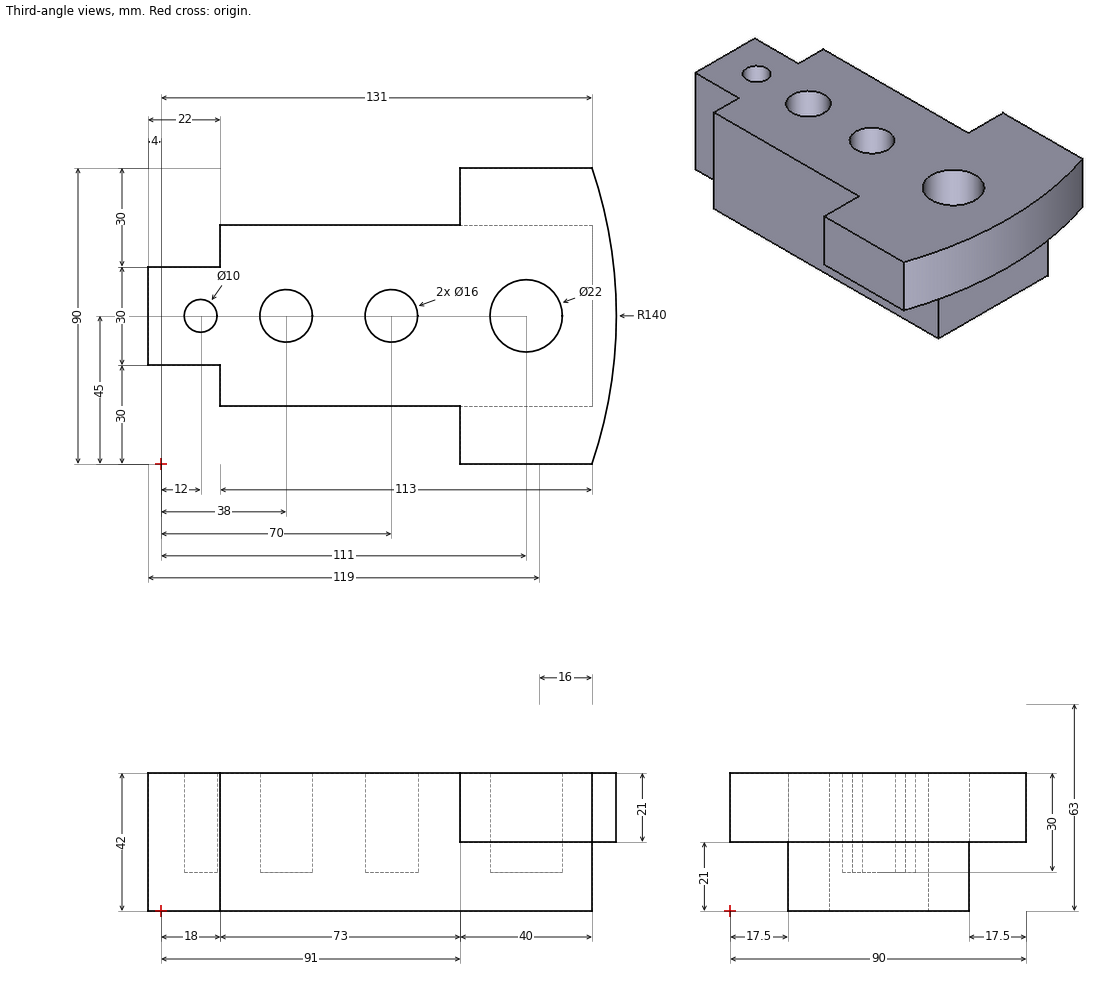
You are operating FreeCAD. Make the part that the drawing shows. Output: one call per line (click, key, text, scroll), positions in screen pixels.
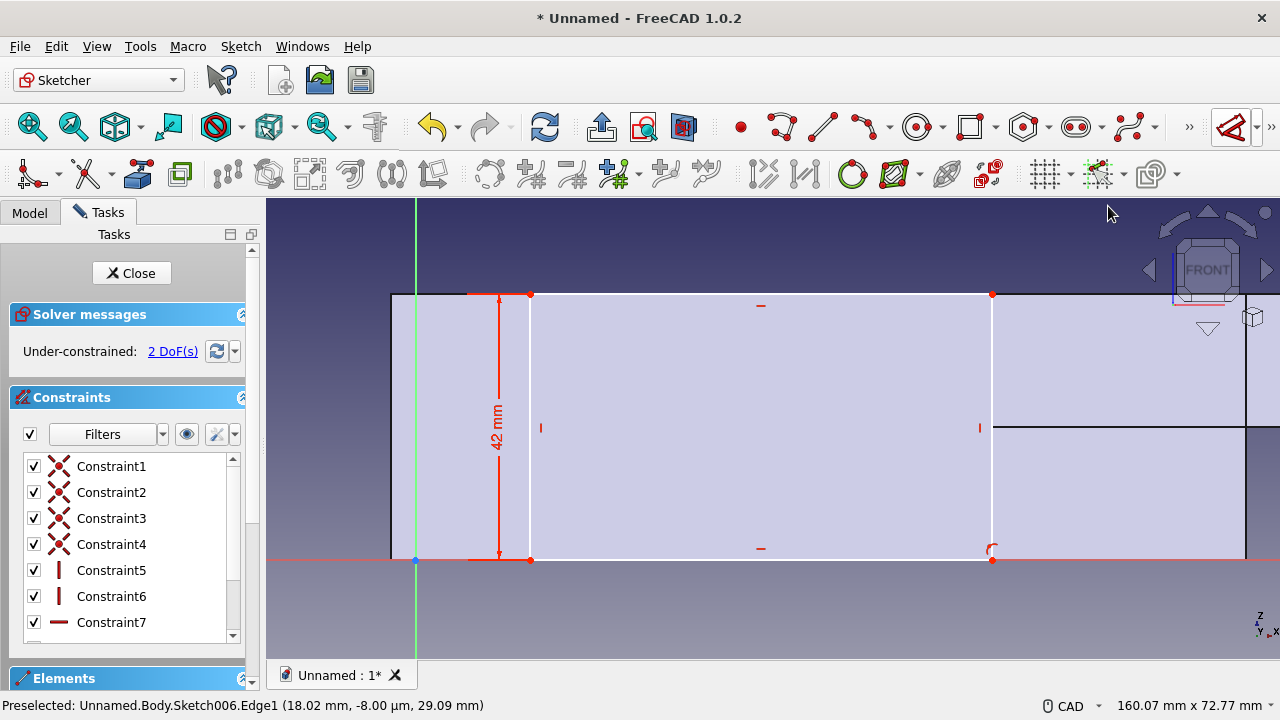
click(669, 560)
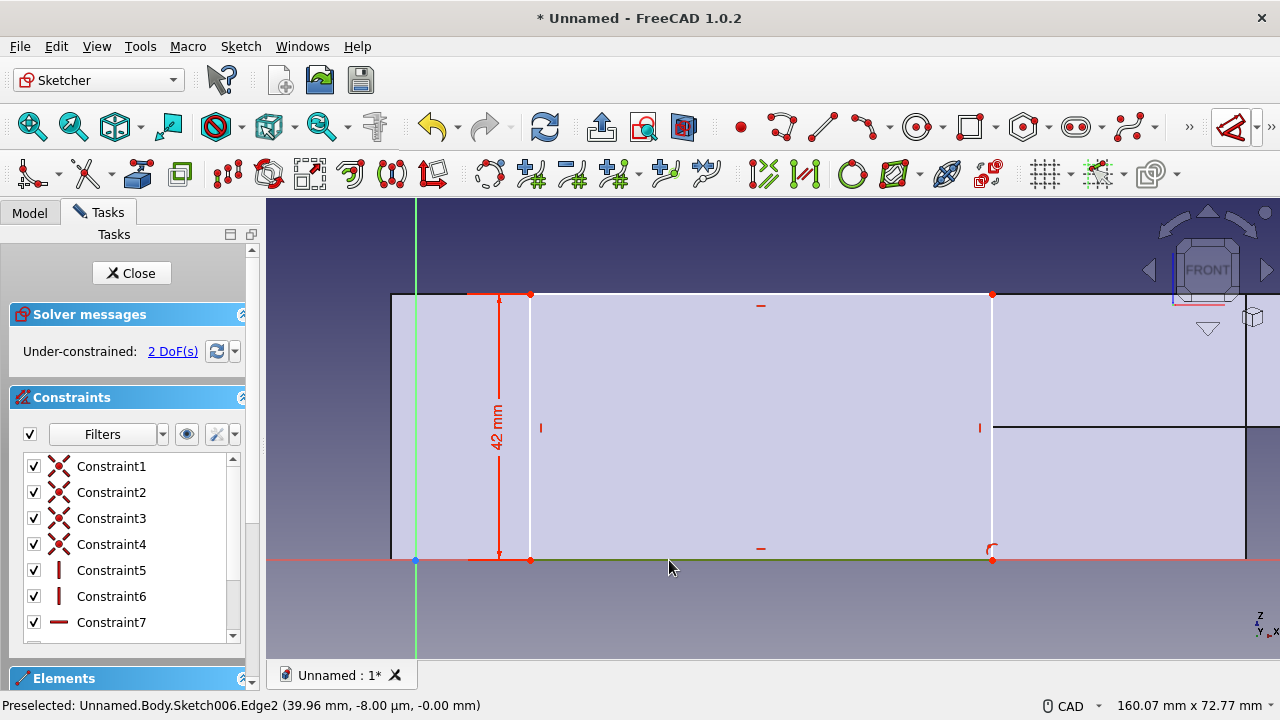
key(l)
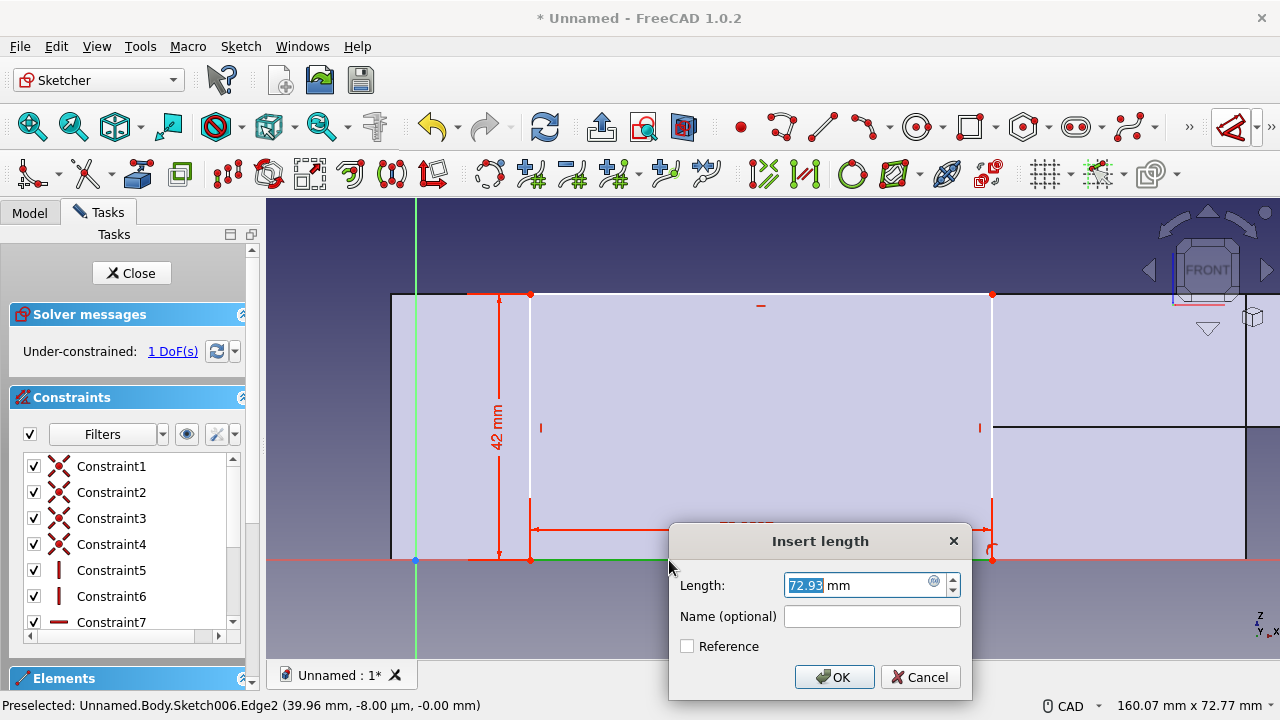
text(73)
key(Return)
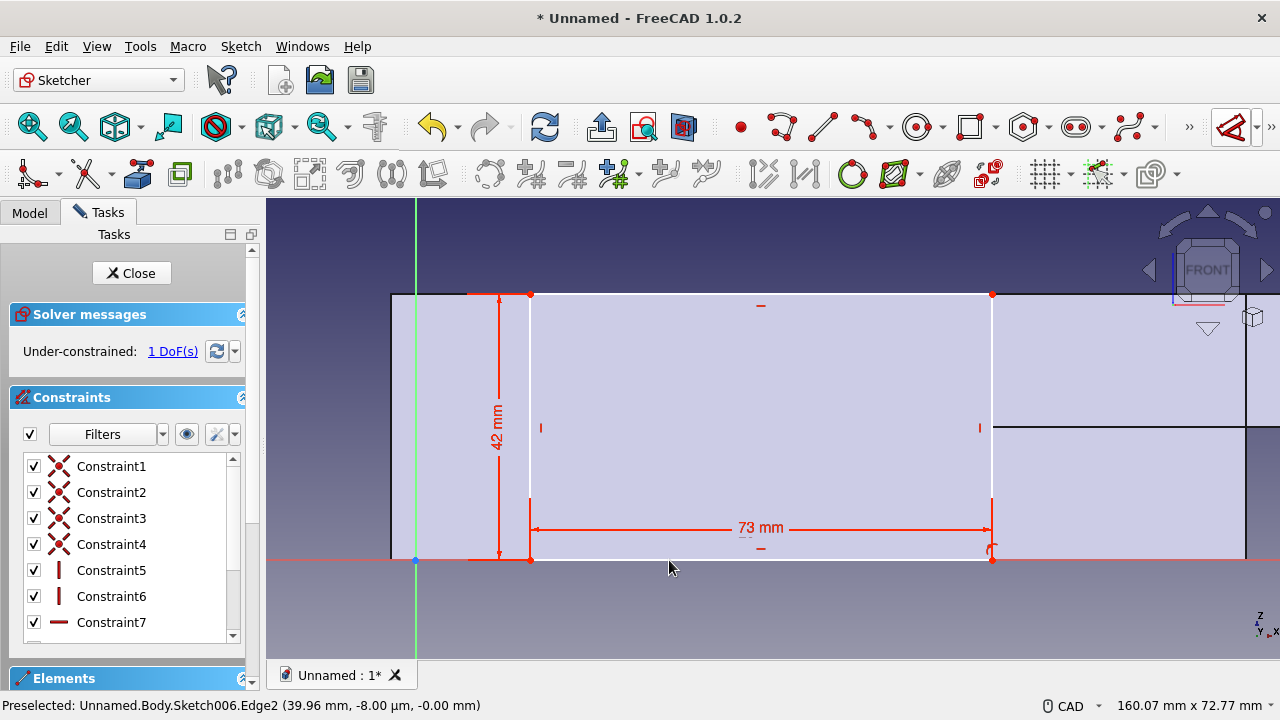
click(530, 294)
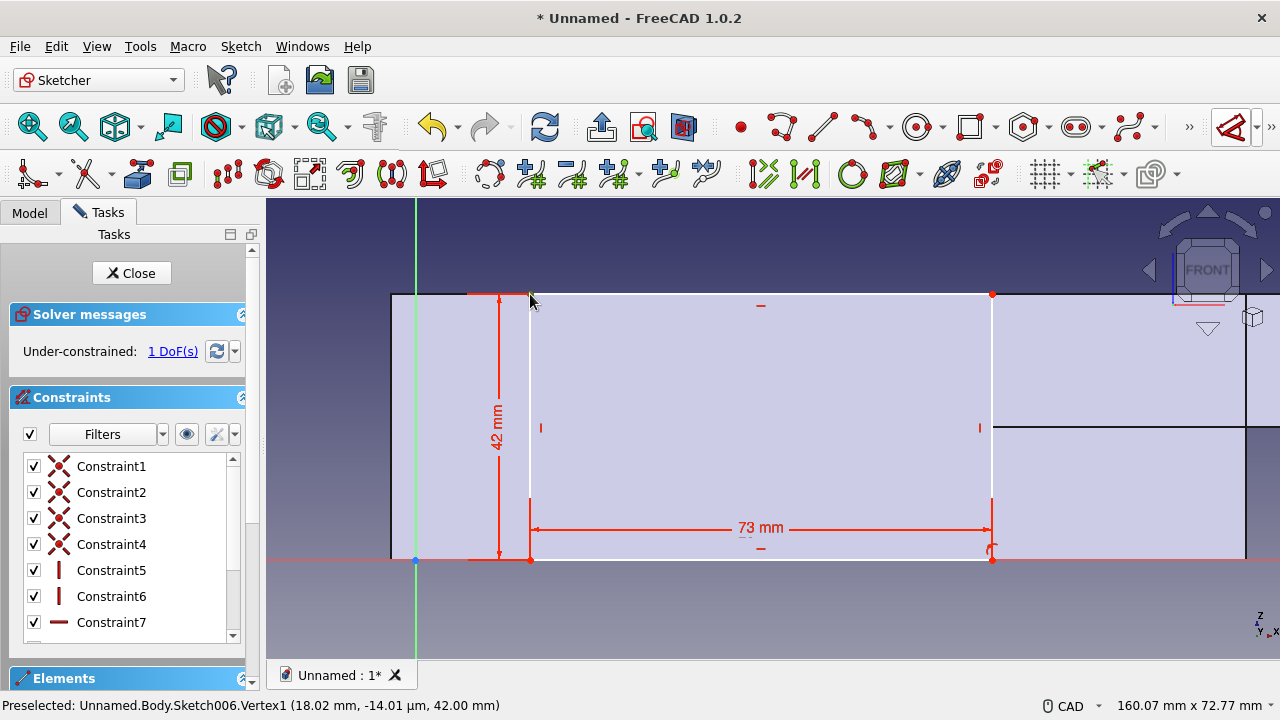
click(1256, 128)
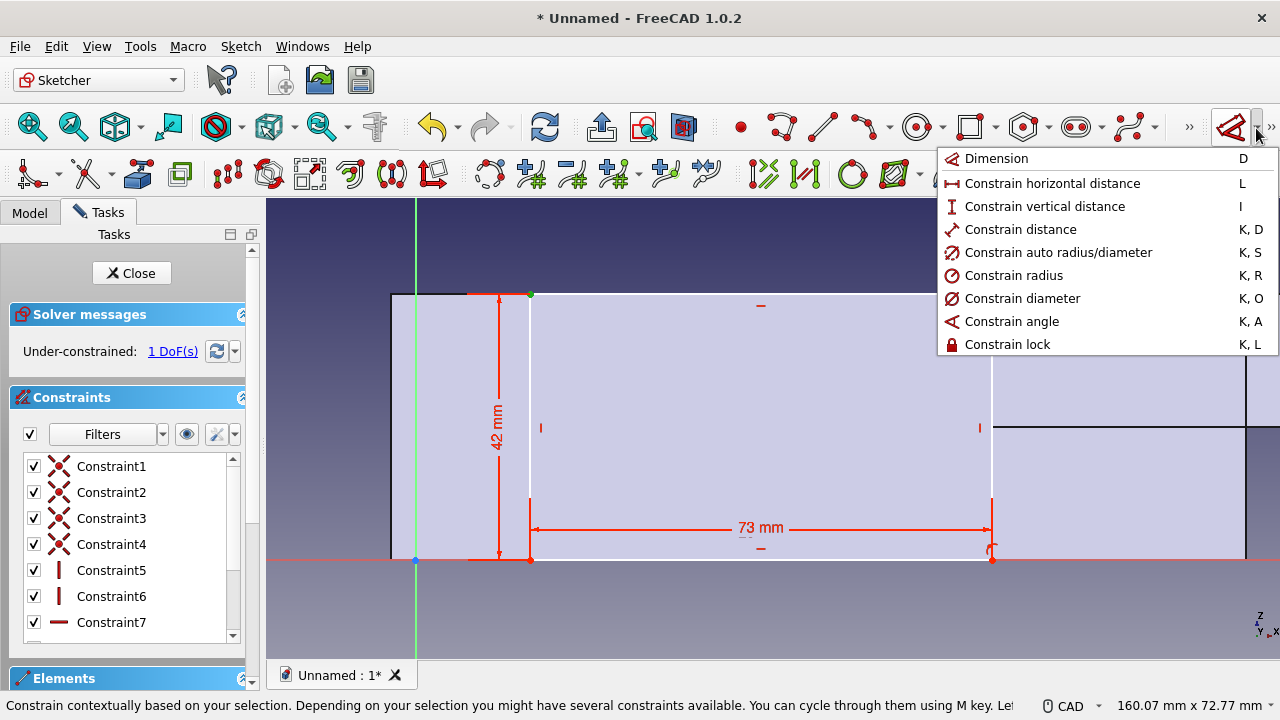
click(1108, 184)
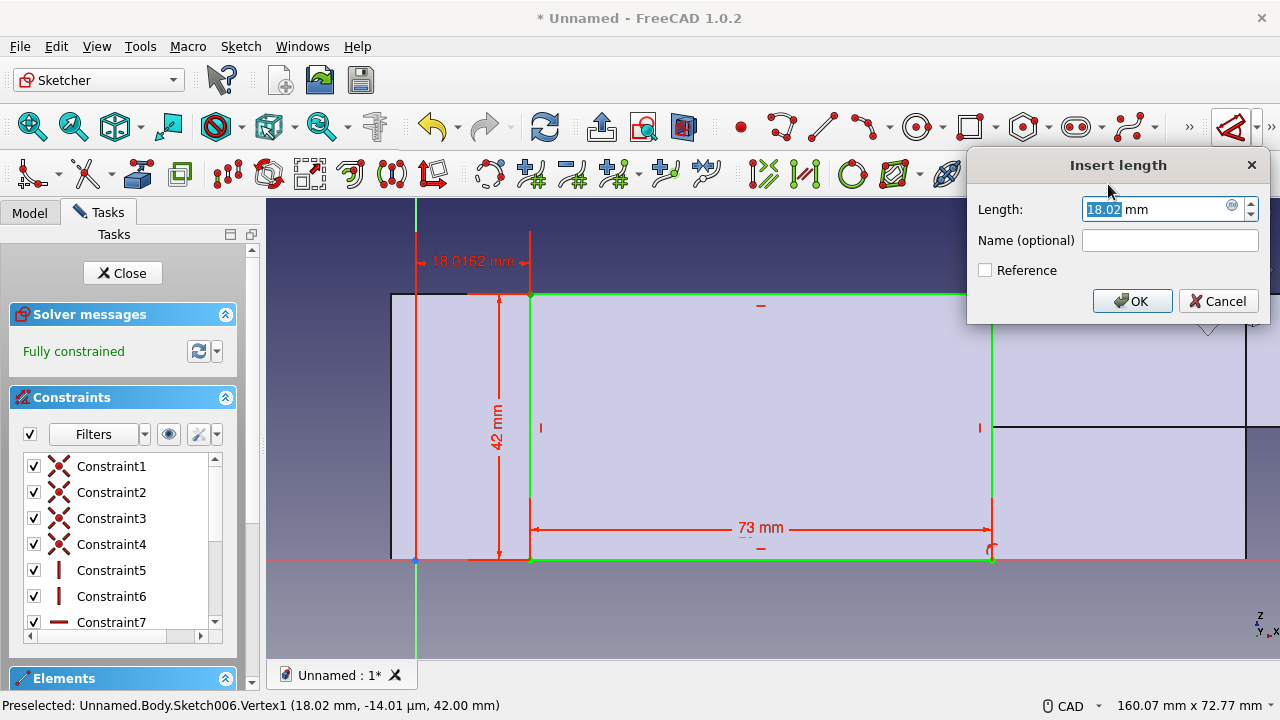
text(18)
key(Return)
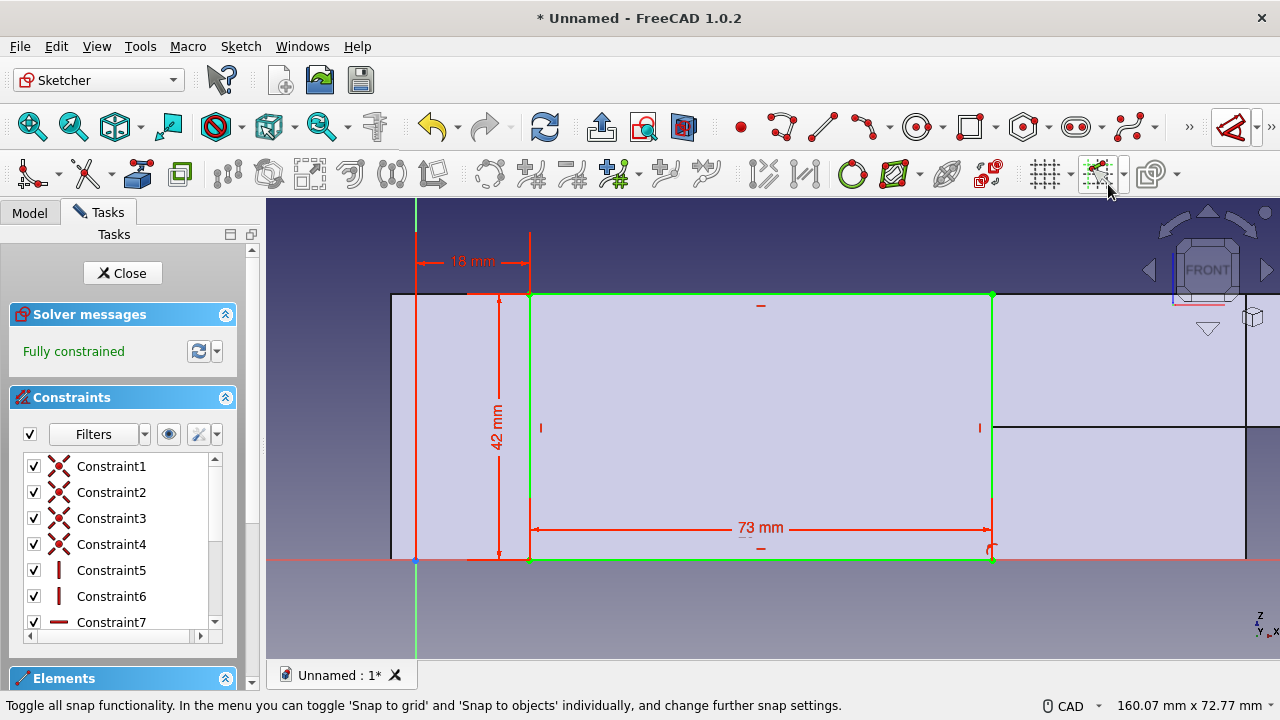
click(123, 273)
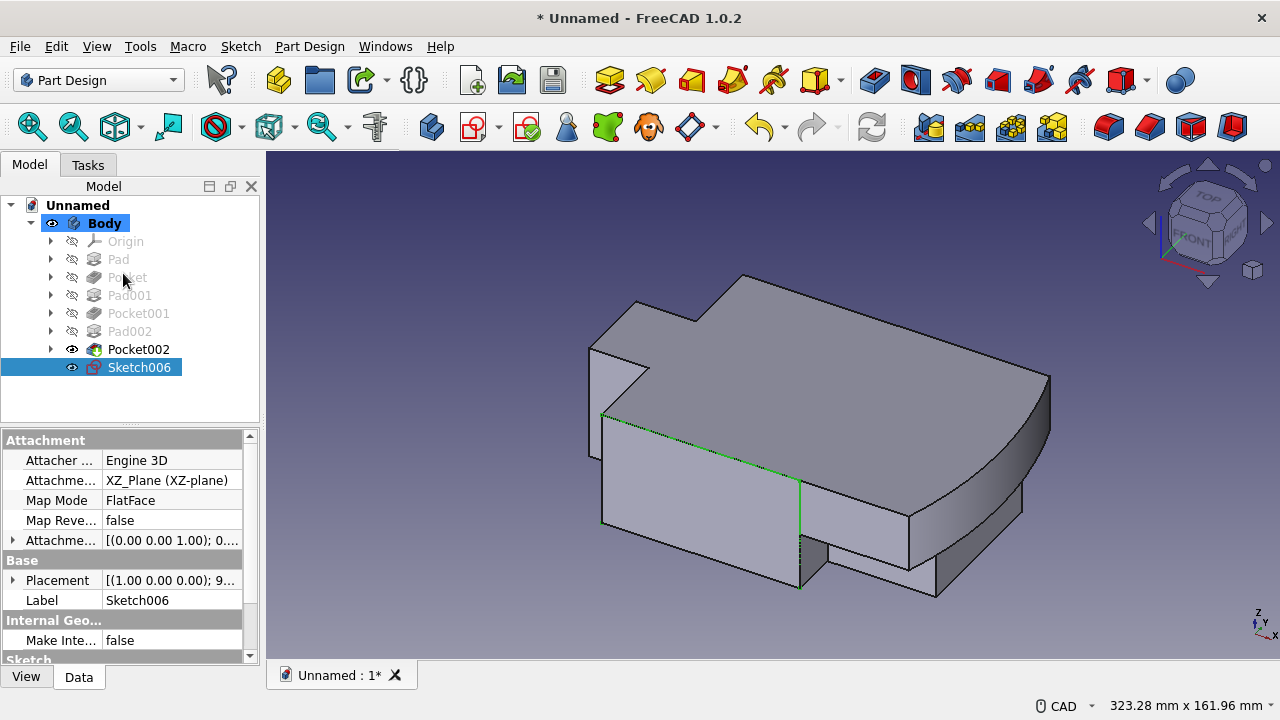
click(875, 80)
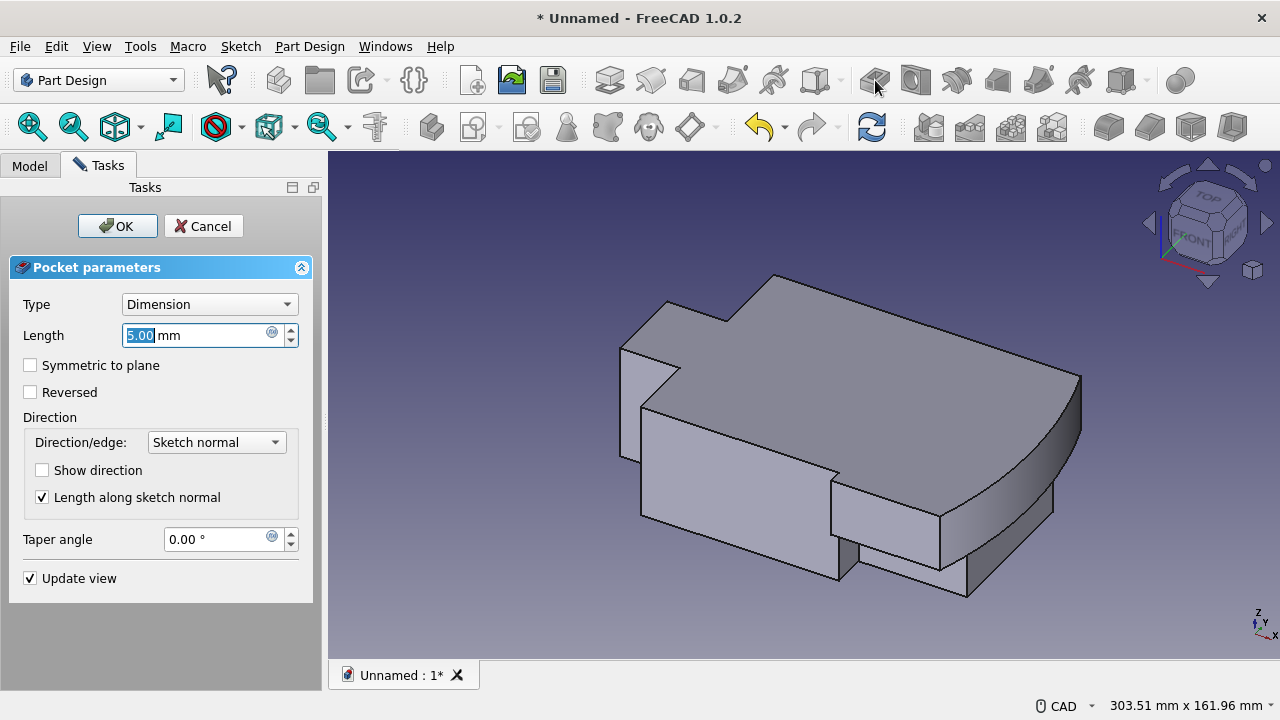
text(17.5)
key(Tab)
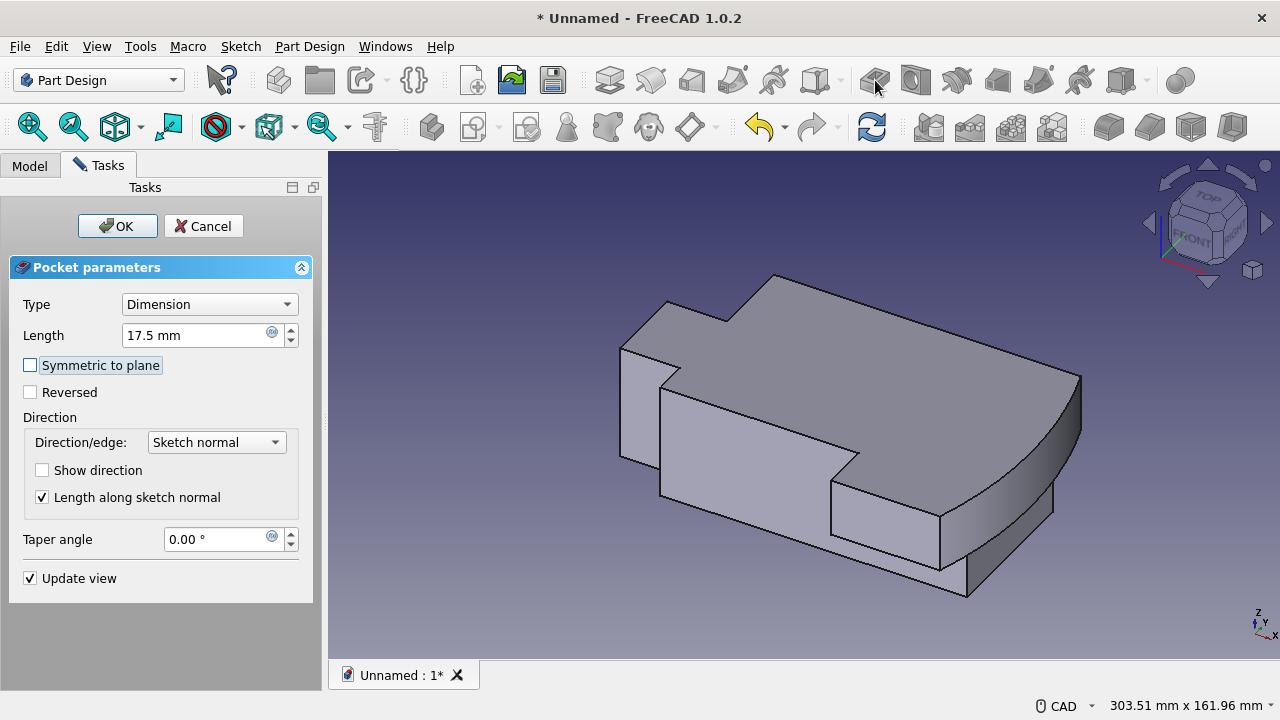
click(118, 226)